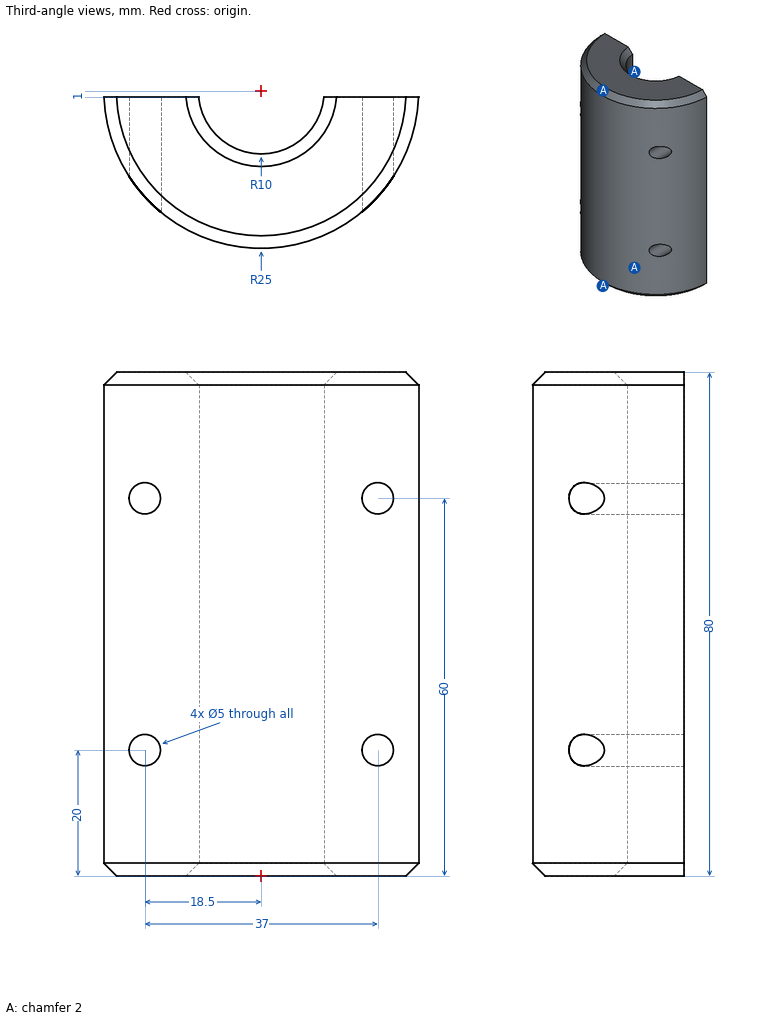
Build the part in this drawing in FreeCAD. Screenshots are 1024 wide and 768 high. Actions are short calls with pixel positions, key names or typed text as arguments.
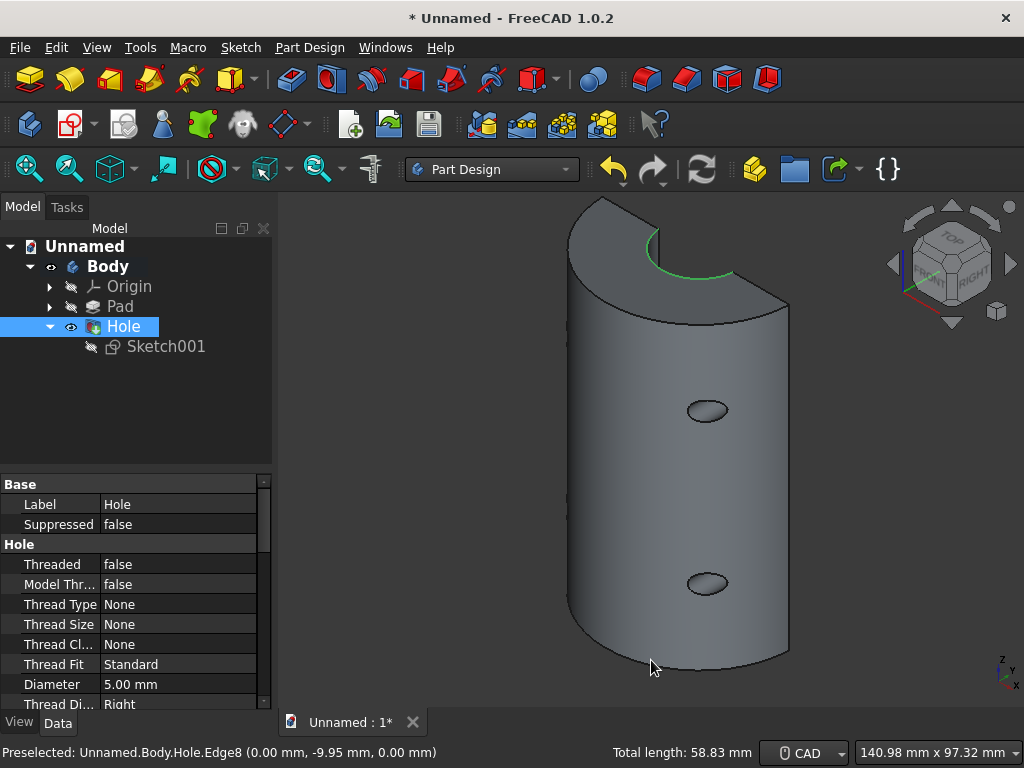
click(606, 302, ctrl)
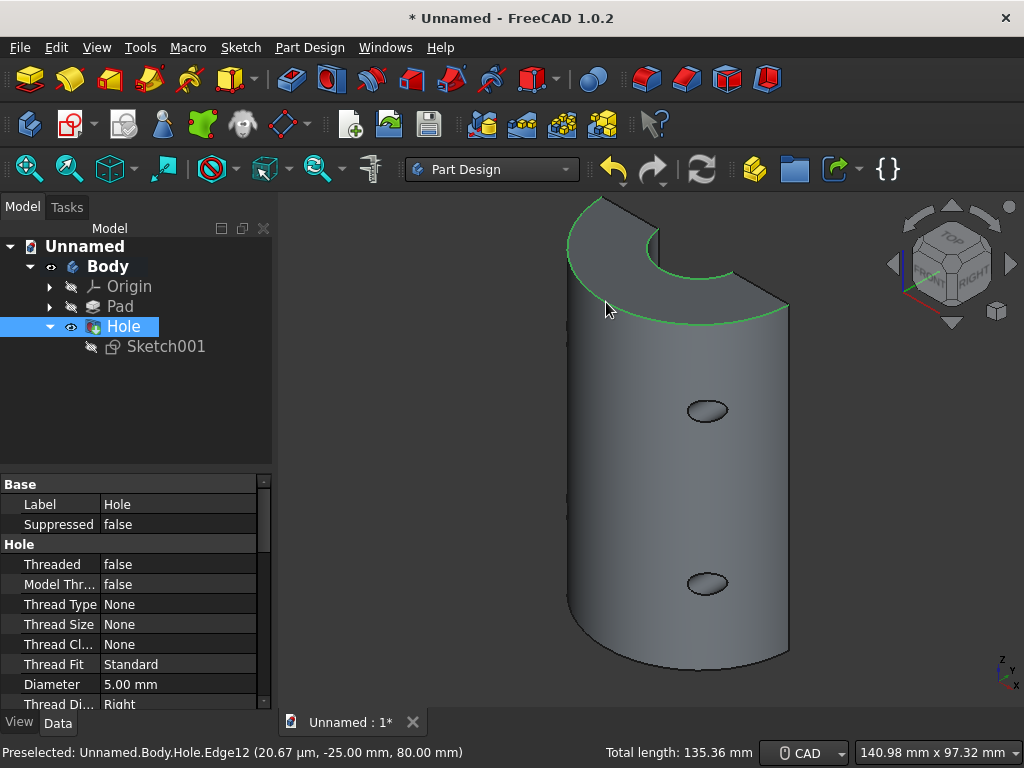
key(2)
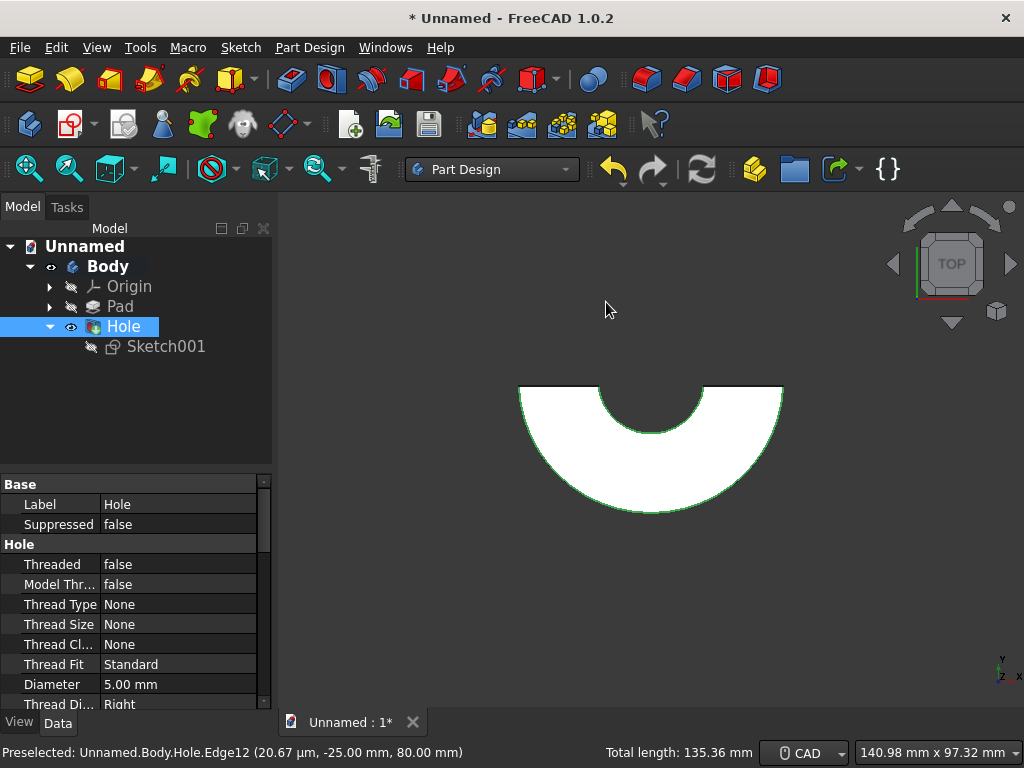
click(30, 170)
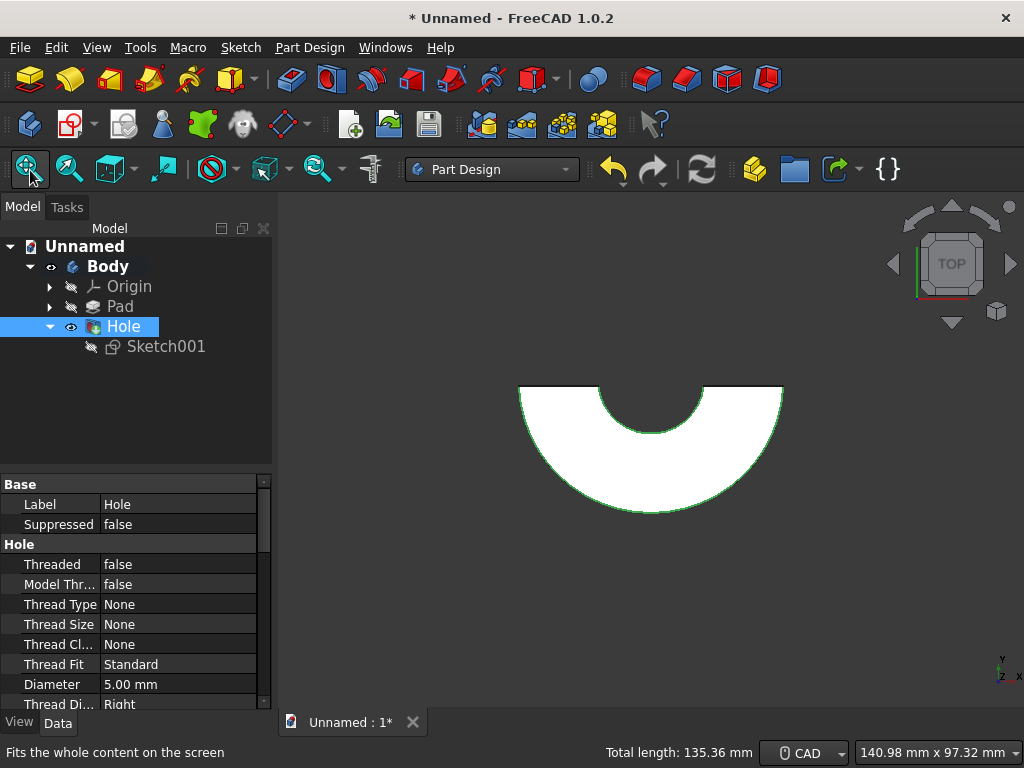
key(1)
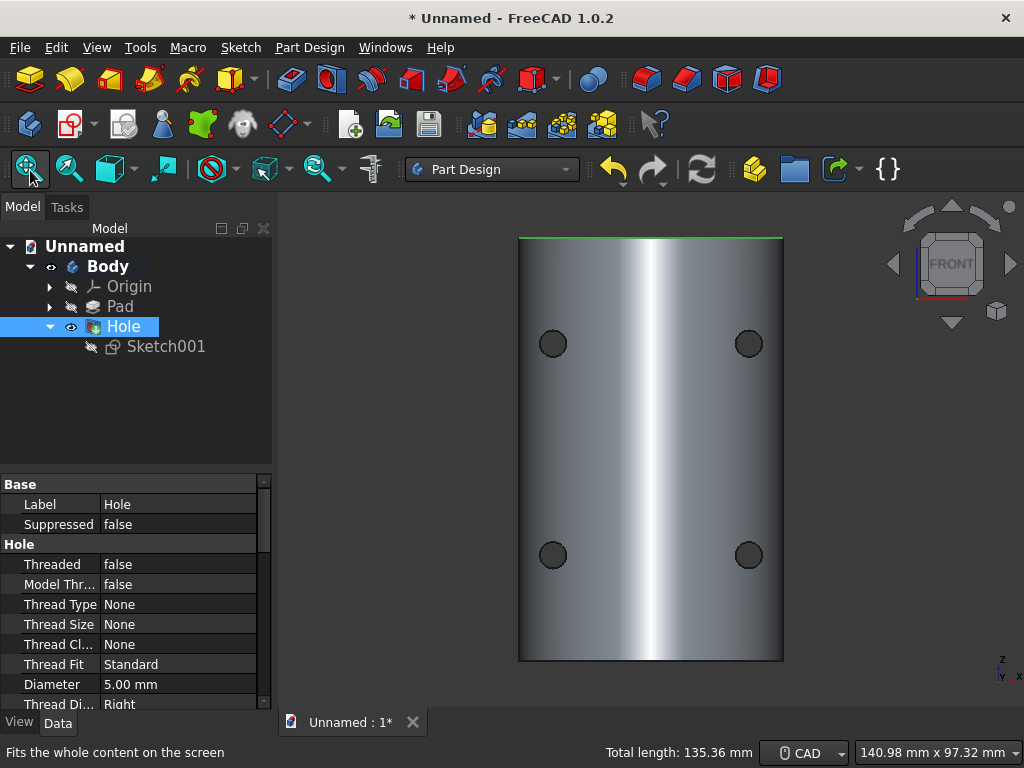
click(651, 660, ctrl)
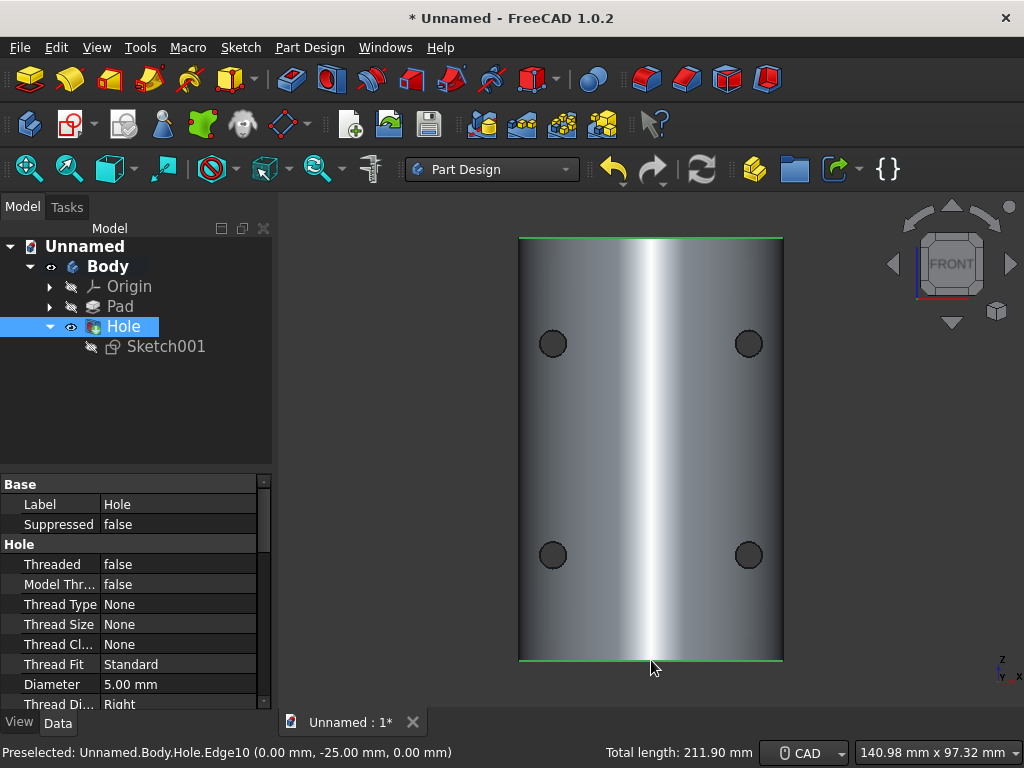
click(688, 80)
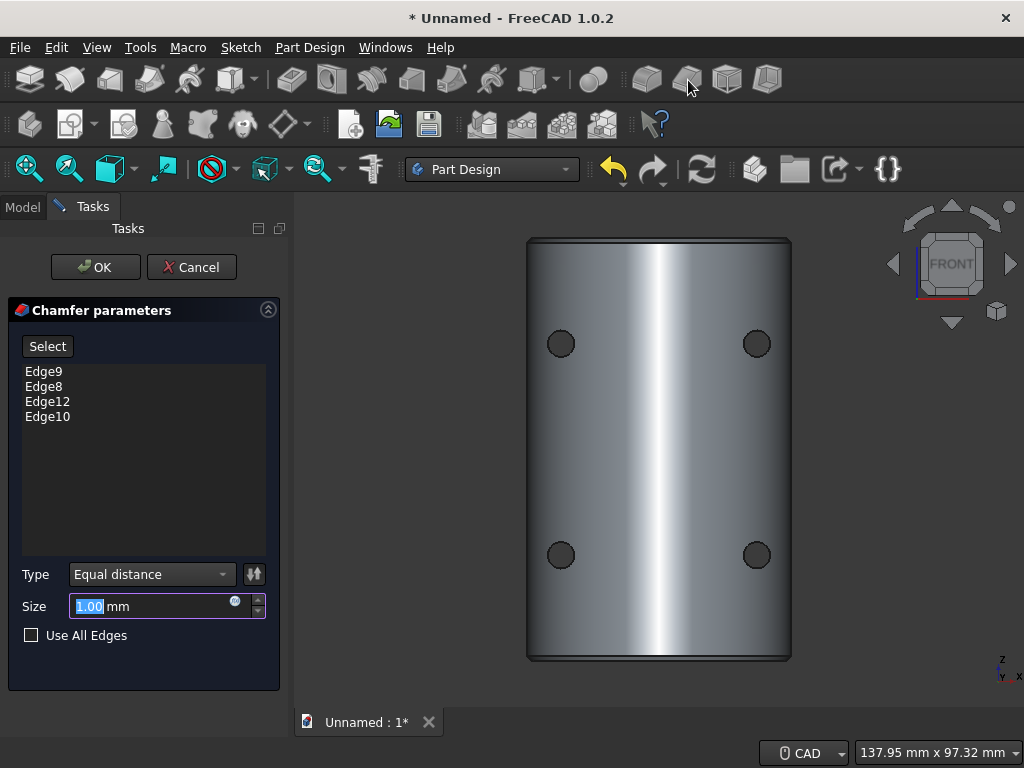
text(2)
key(Tab)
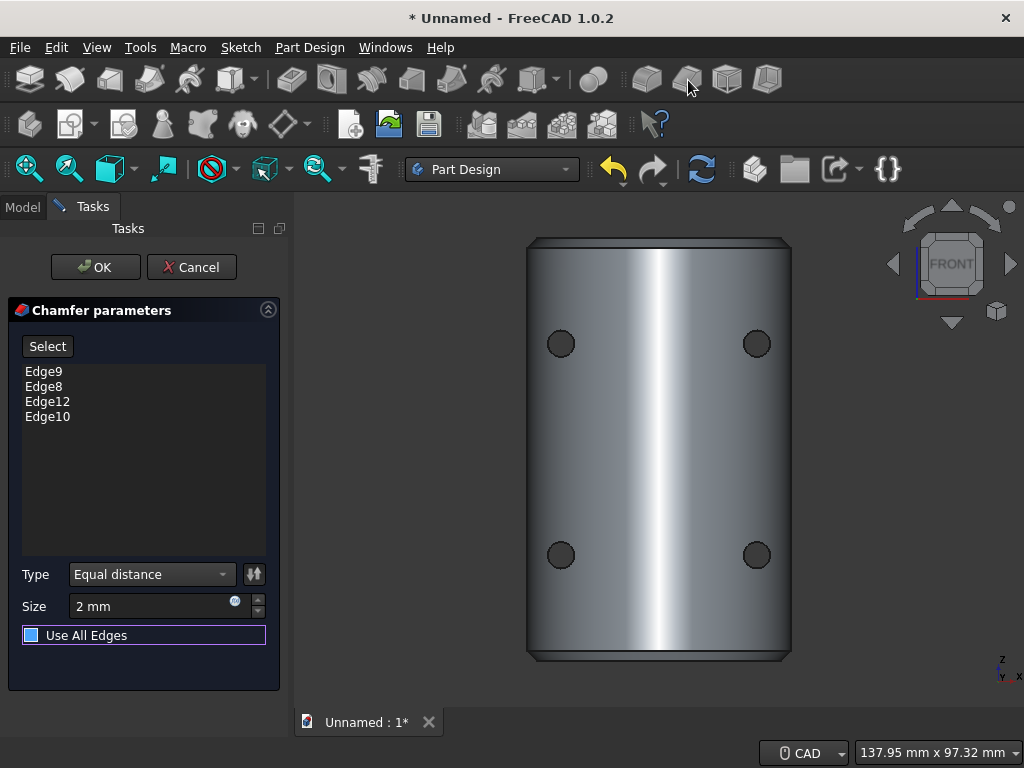
click(96, 267)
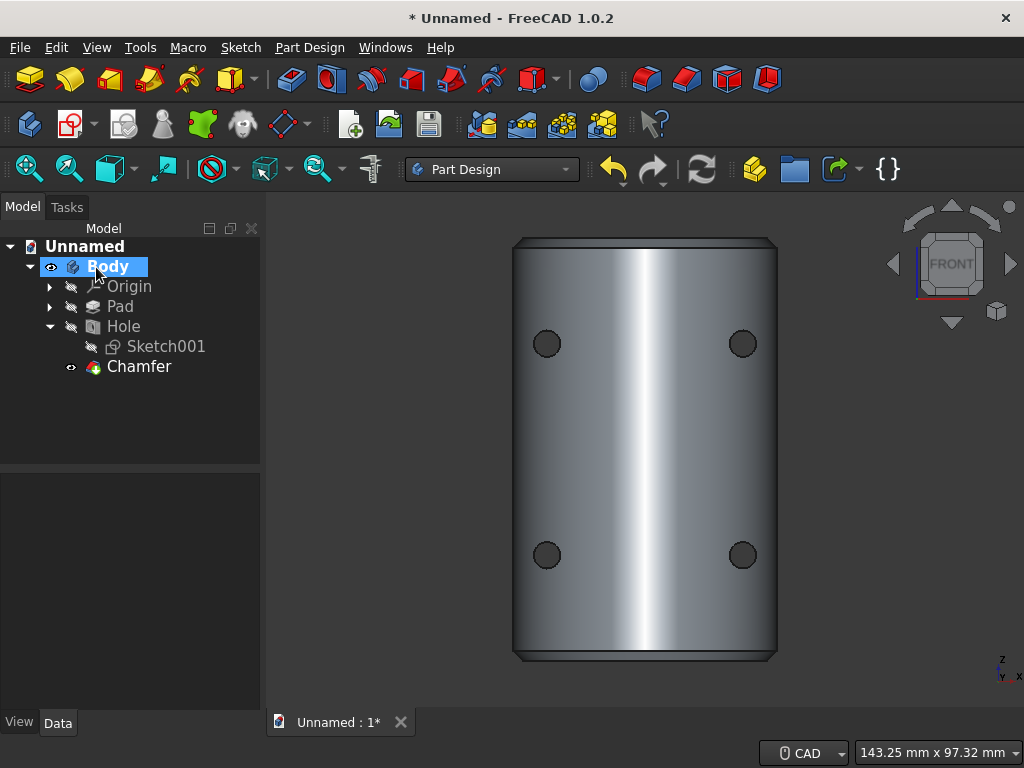
key(0)